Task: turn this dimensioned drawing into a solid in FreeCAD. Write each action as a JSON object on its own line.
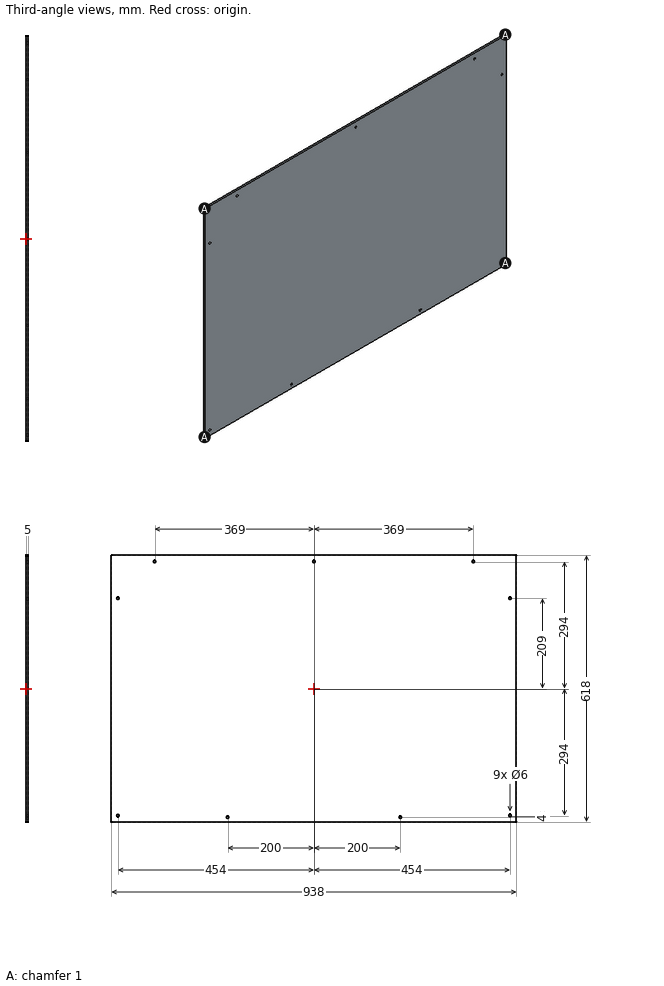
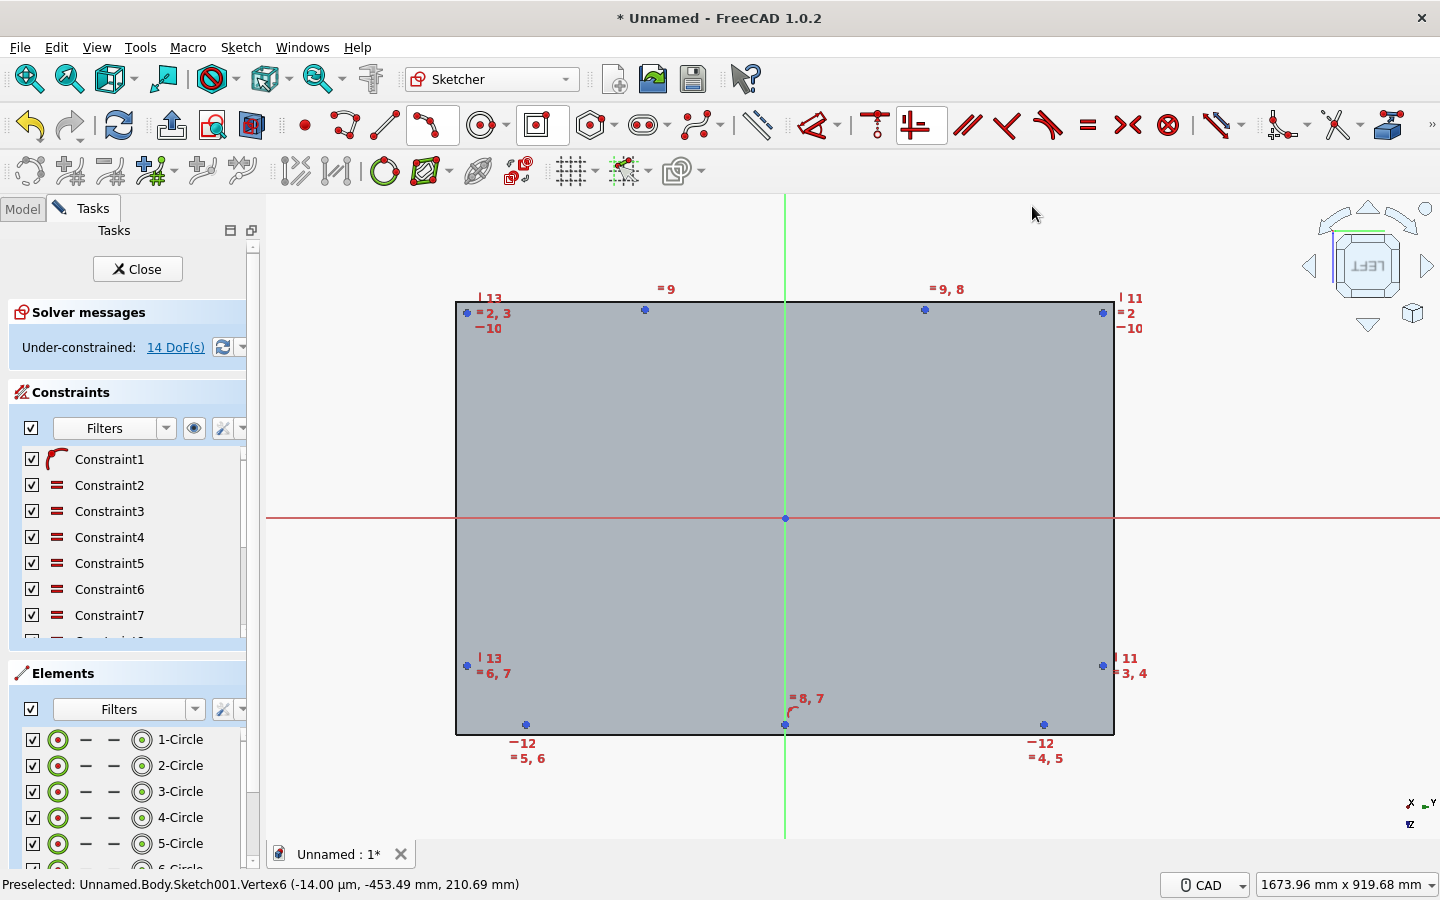
{"action": "left_click", "coordinate": [1103, 666]}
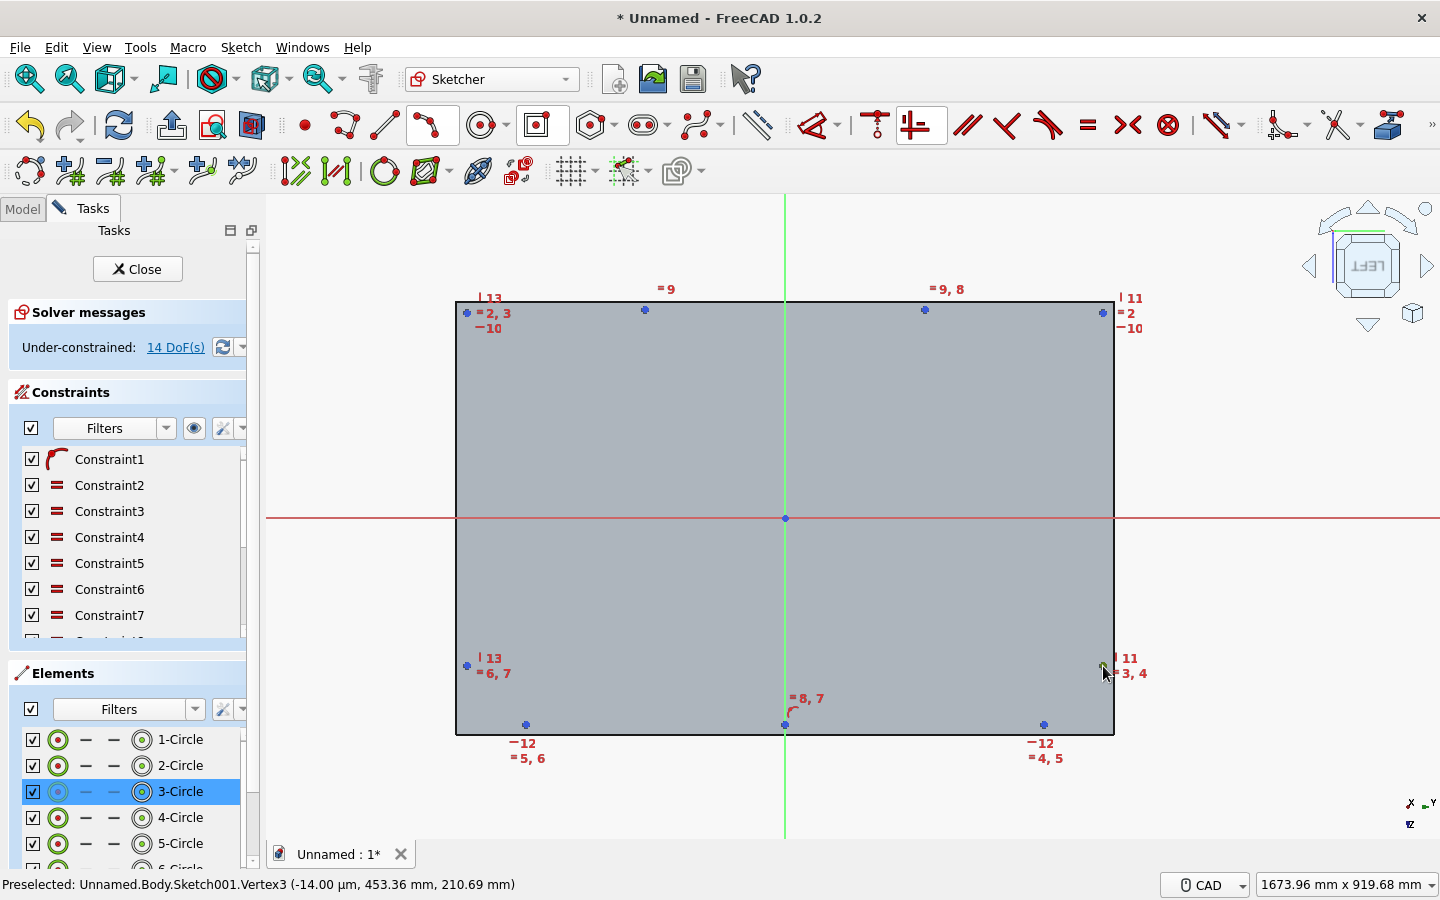
{"action": "left_click", "coordinate": [467, 666]}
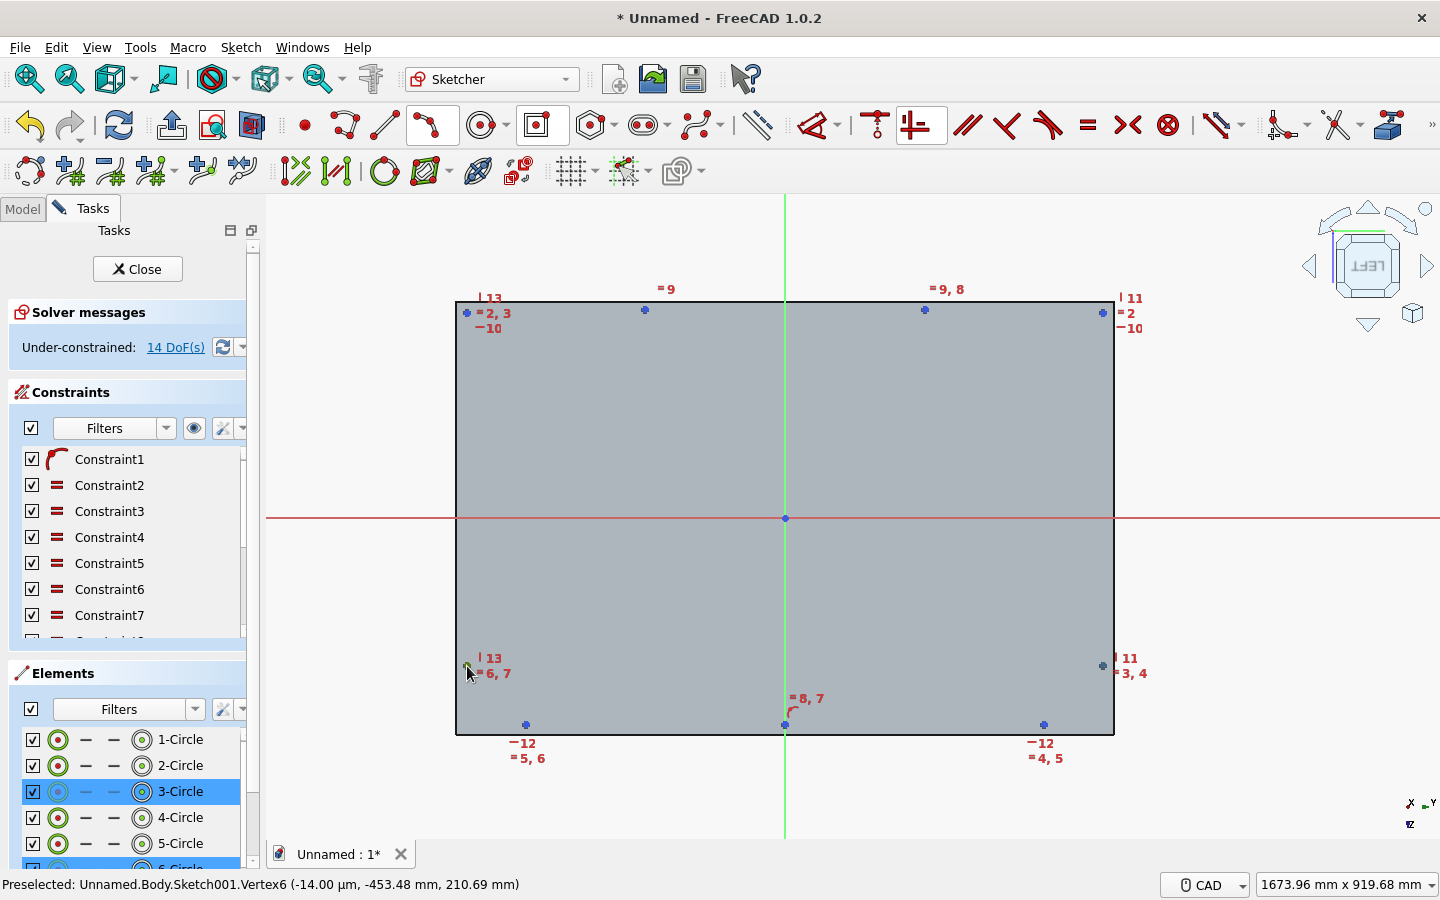
{"action": "left_click", "coordinate": [942, 126]}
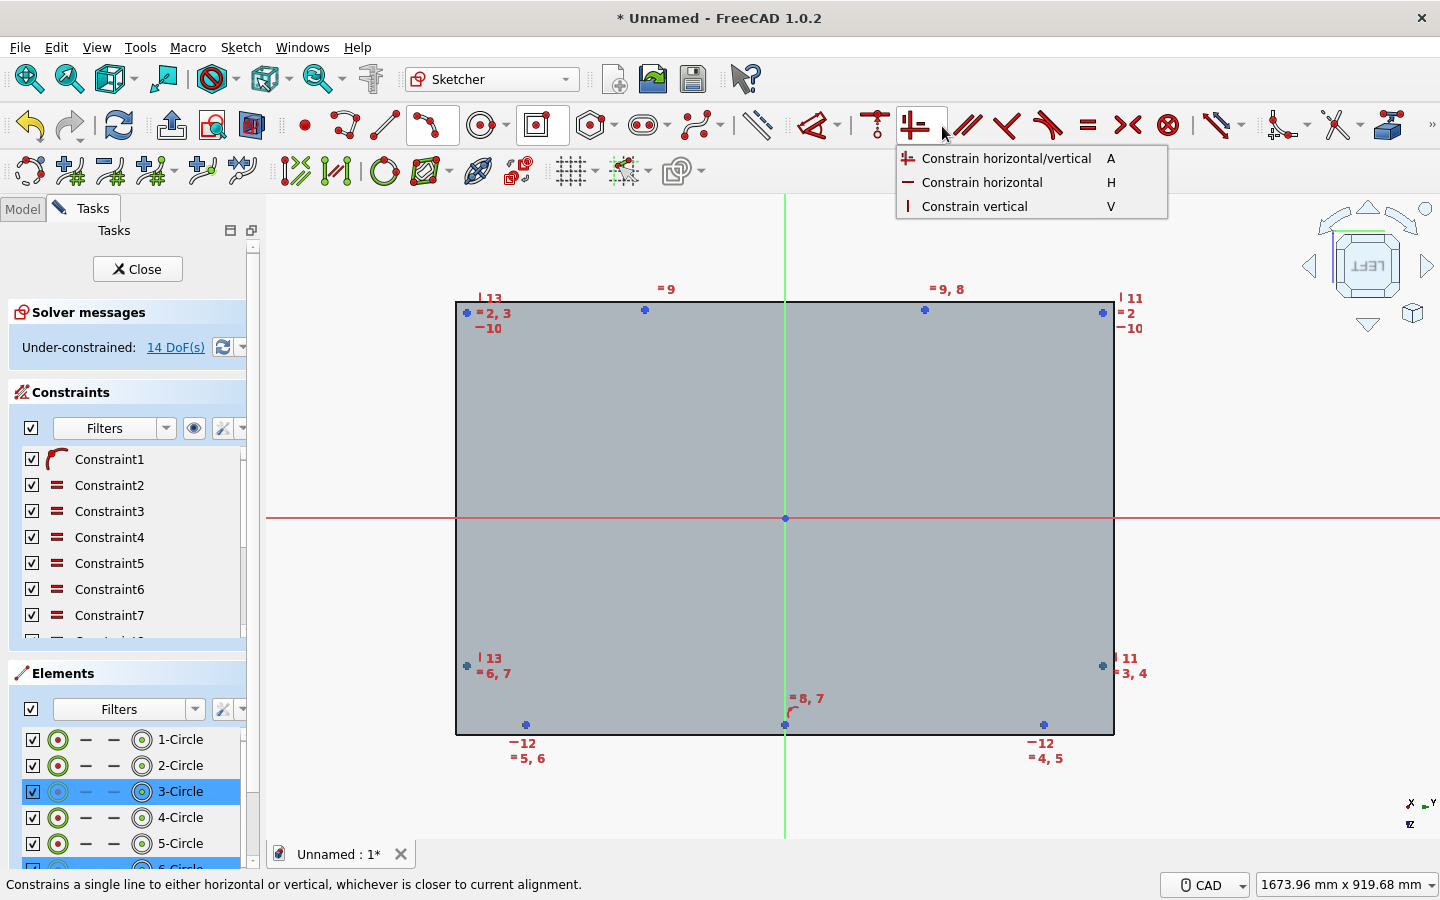
{"action": "left_click", "coordinate": [1032, 182]}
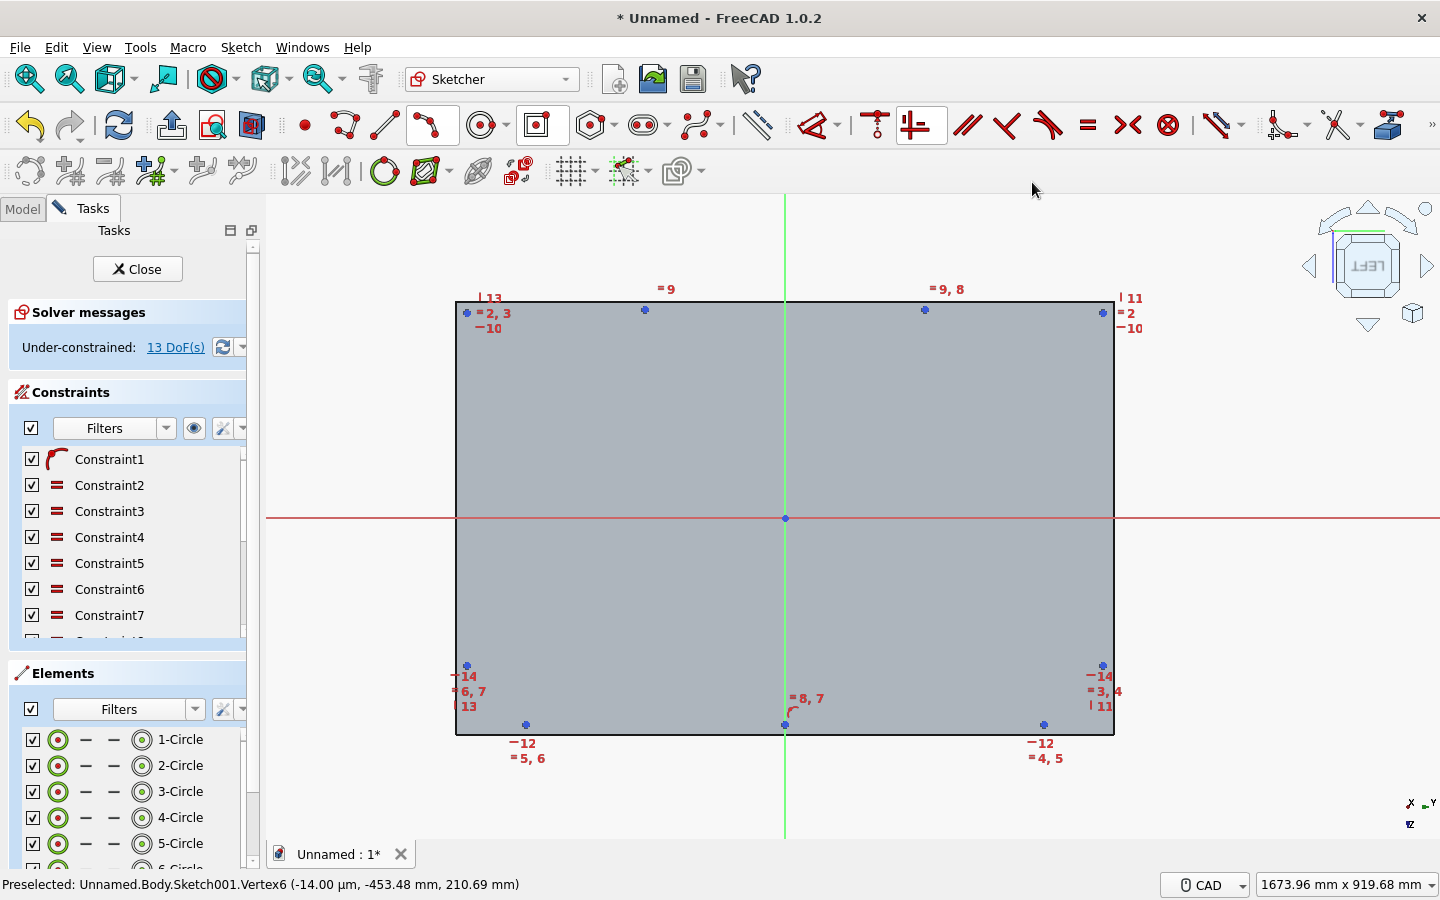
{"action": "left_click", "coordinate": [1044, 725]}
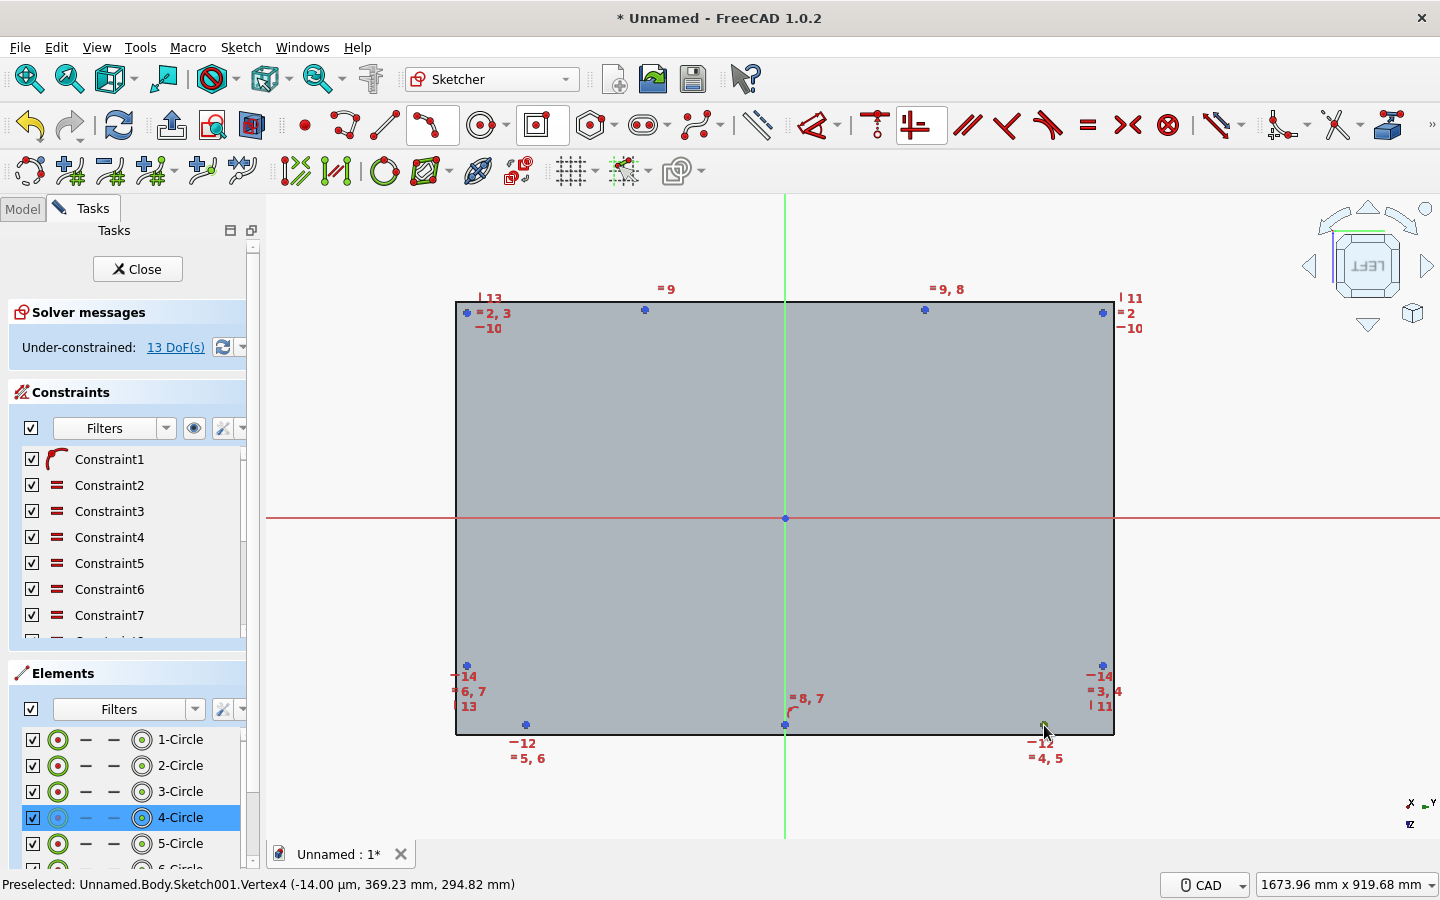
{"action": "left_click", "coordinate": [785, 725]}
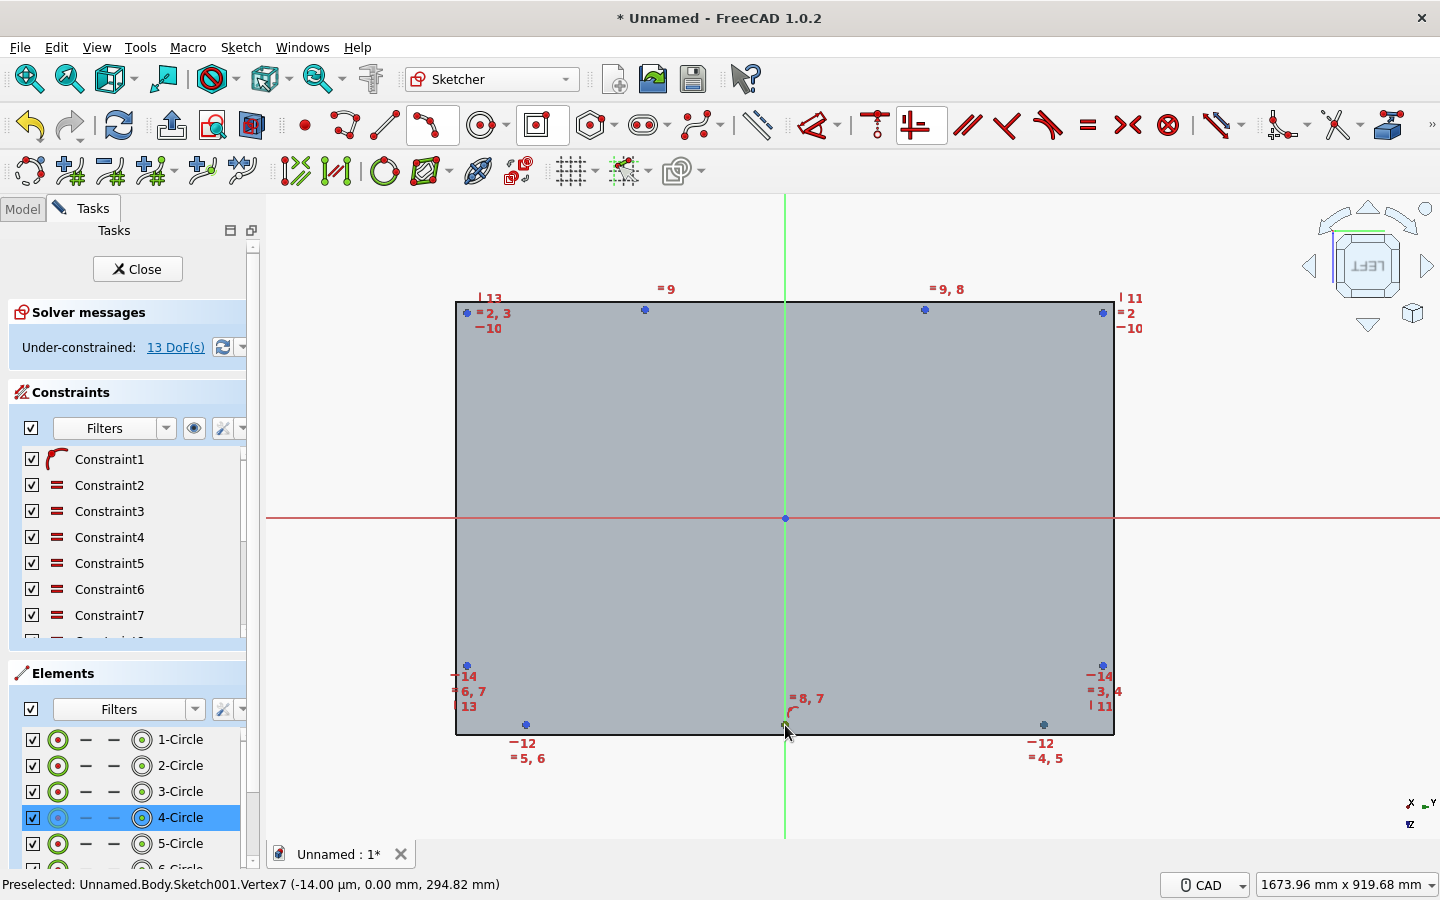
{"action": "left_click", "coordinate": [942, 126]}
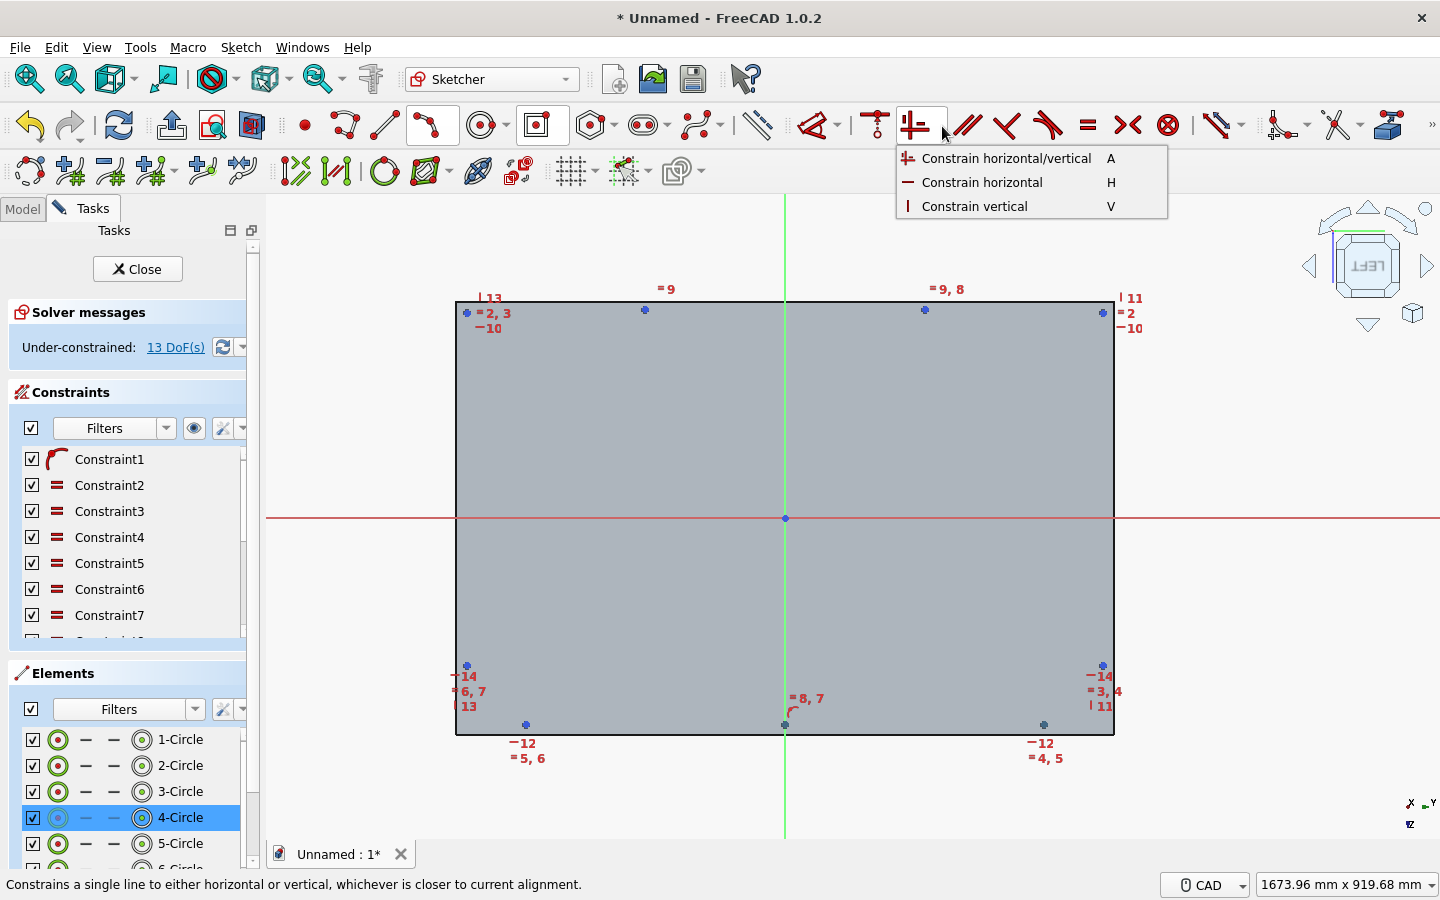
{"action": "left_click", "coordinate": [1032, 182]}